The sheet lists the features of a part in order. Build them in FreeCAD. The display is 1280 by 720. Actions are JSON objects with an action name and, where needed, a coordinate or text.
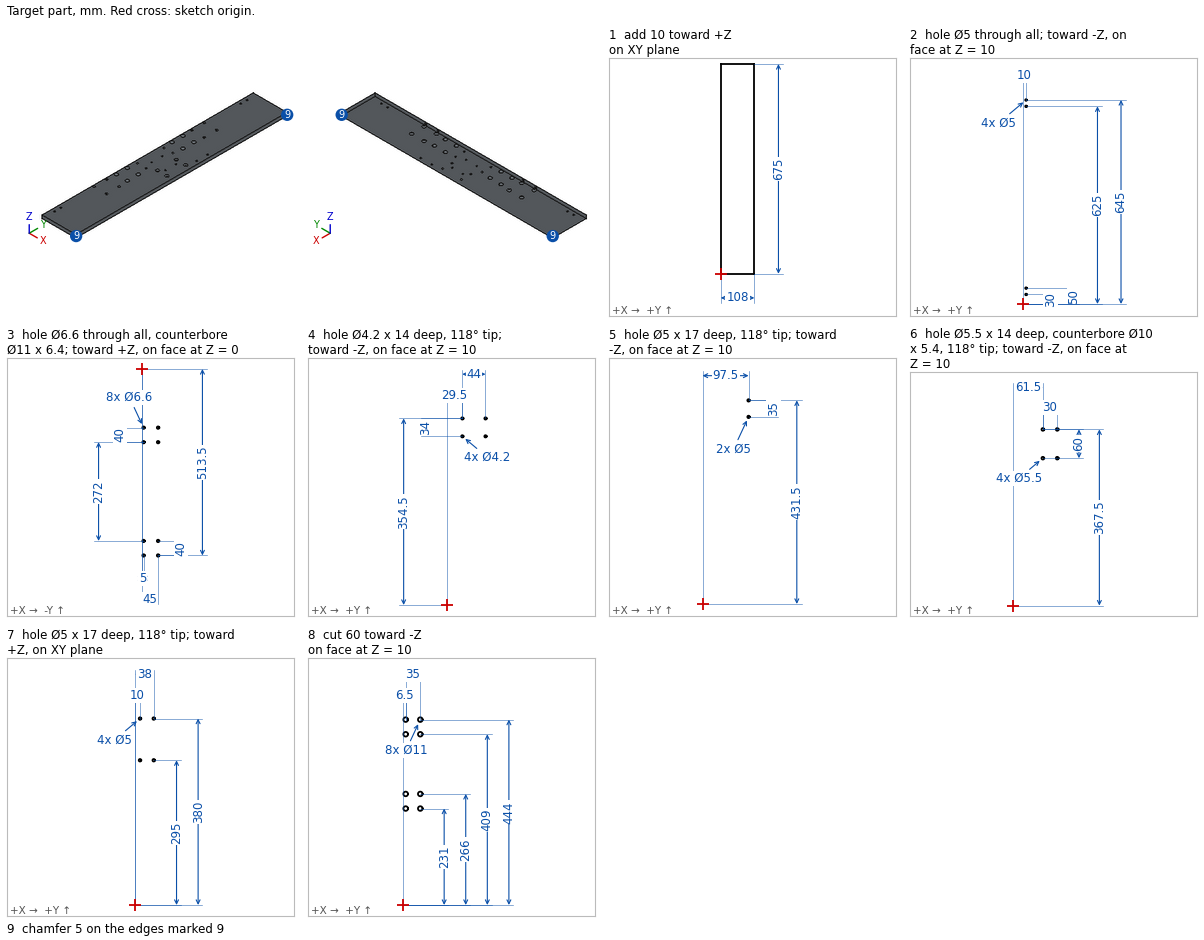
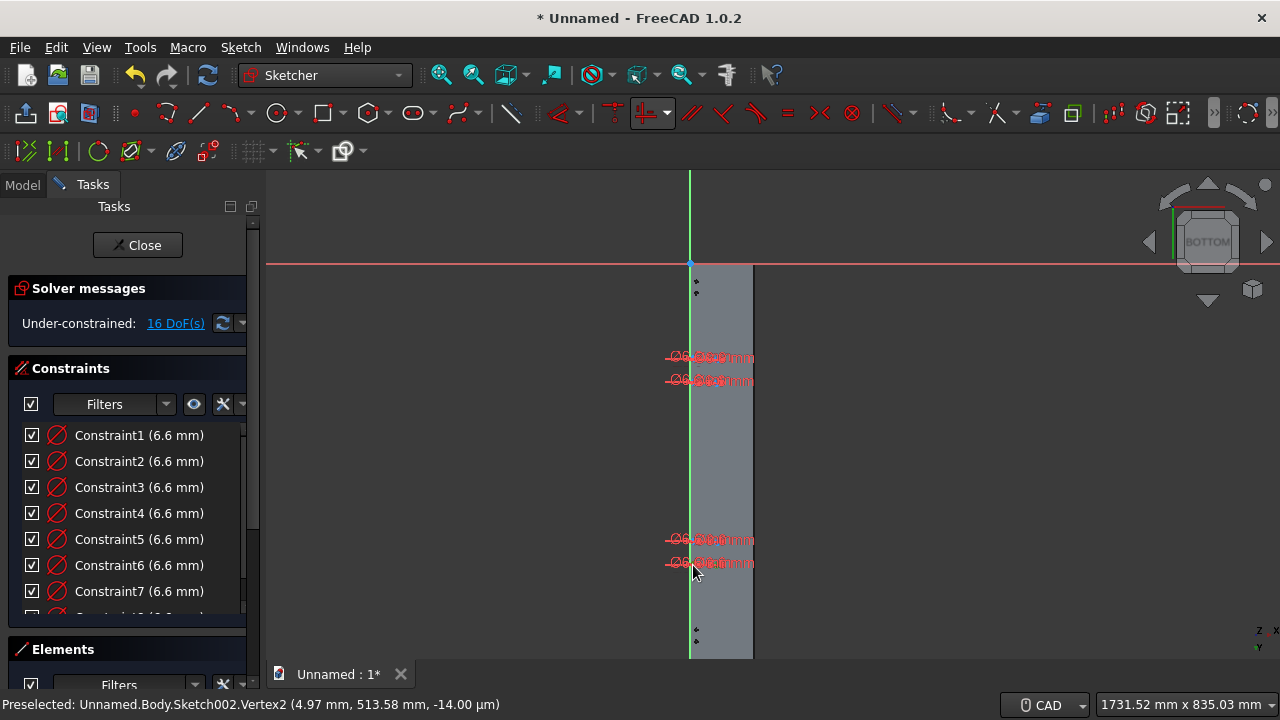
{"action": "key", "text": "h"}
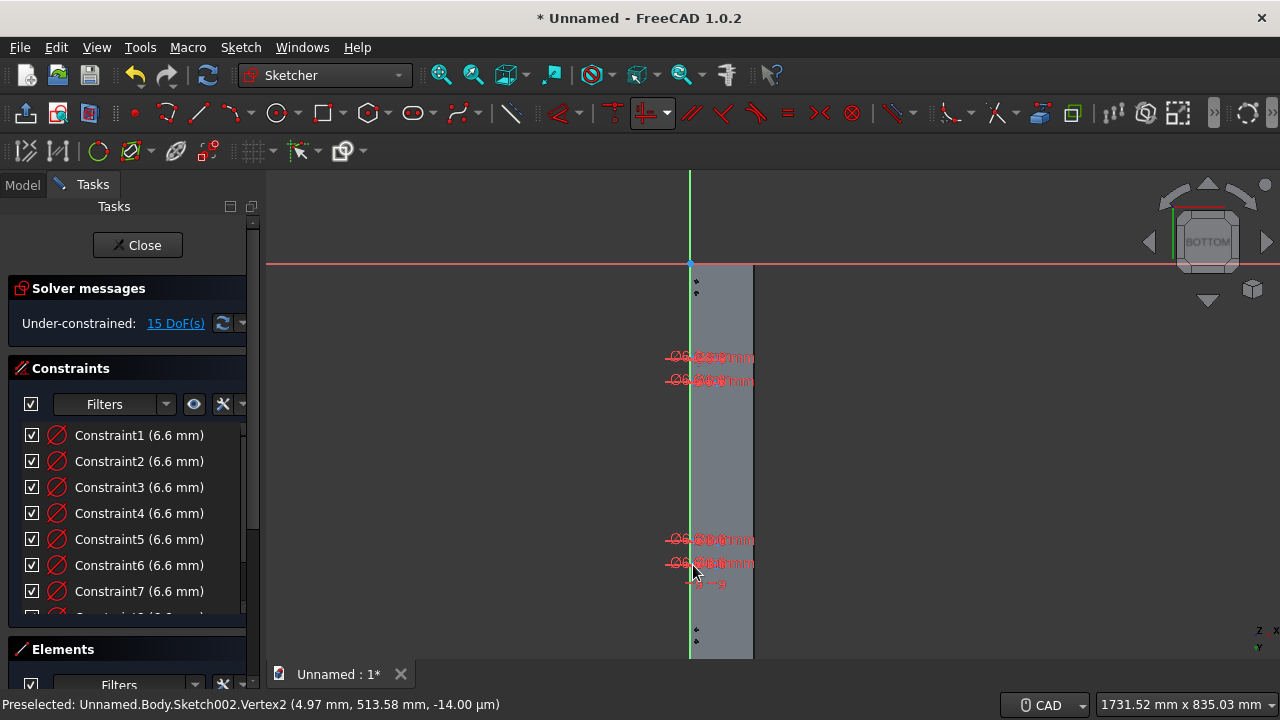
{"action": "left_click", "coordinate": [717, 565]}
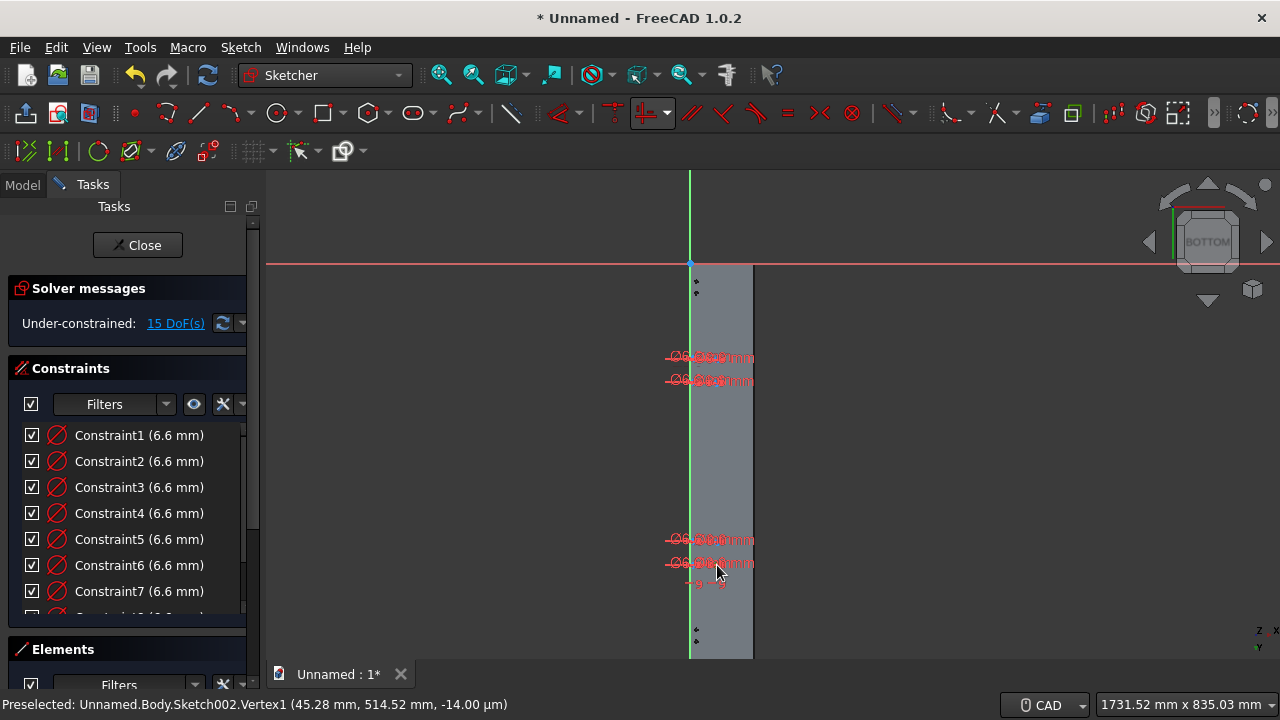
{"action": "left_click", "coordinate": [717, 542]}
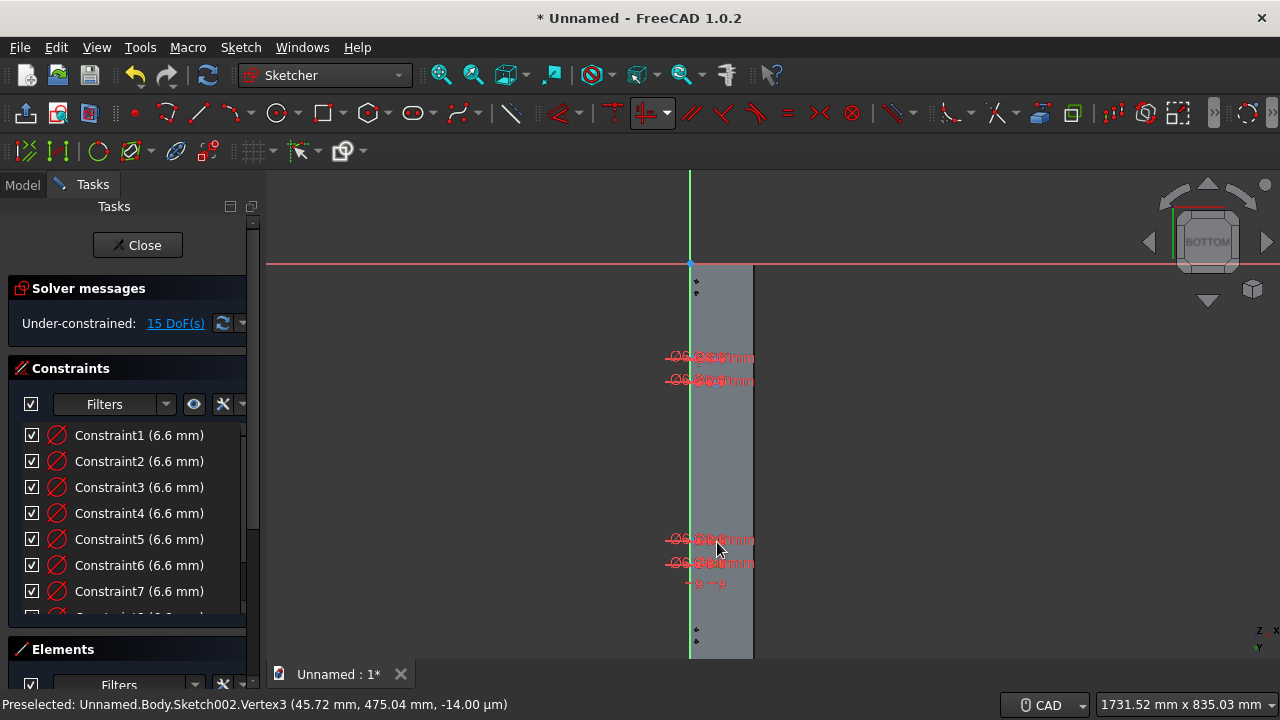
{"action": "key", "text": "v"}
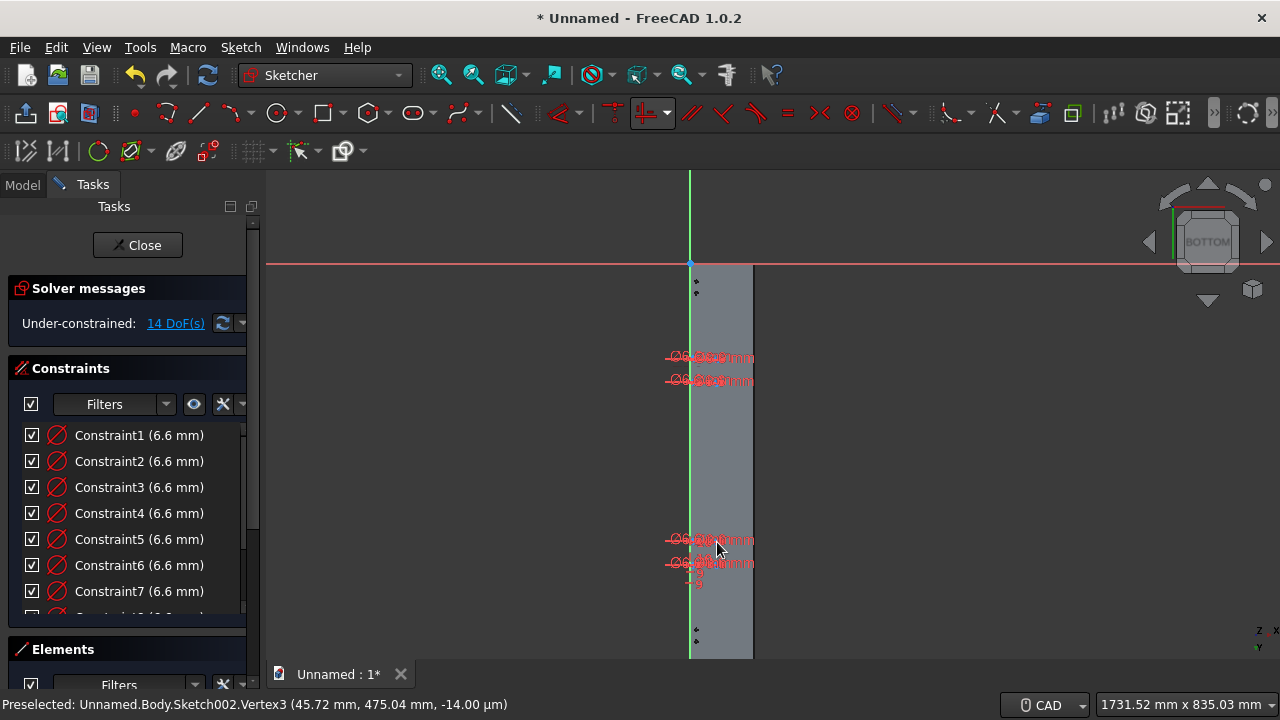
{"action": "left_click", "coordinate": [693, 565]}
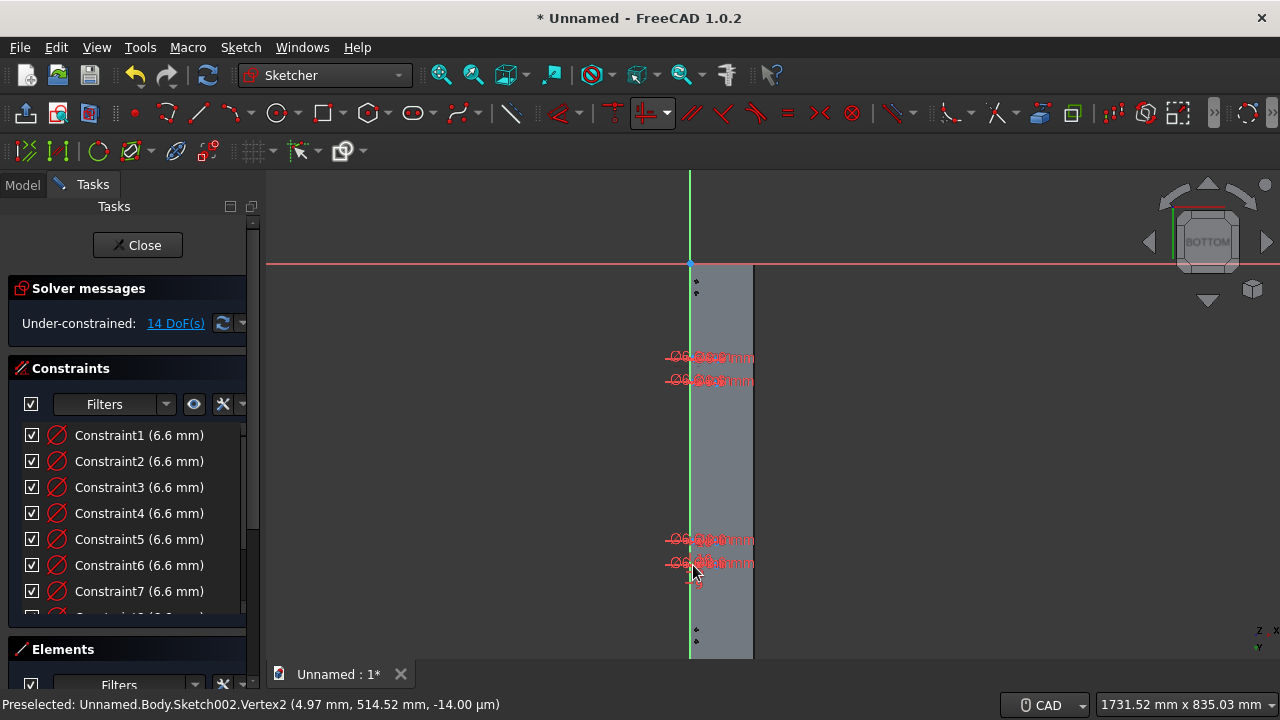
{"action": "scroll", "coordinate": [693, 541], "scroll_direction": "up", "scroll_amount": 4}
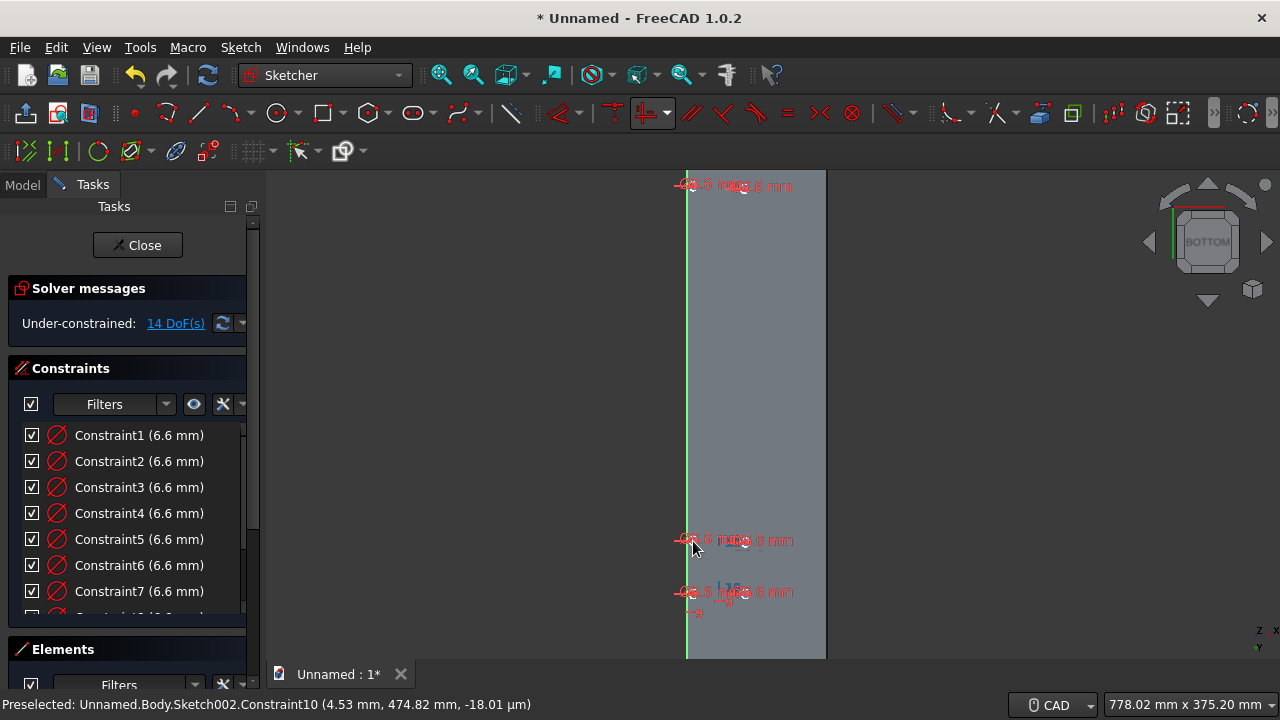
{"action": "left_click", "coordinate": [693, 541]}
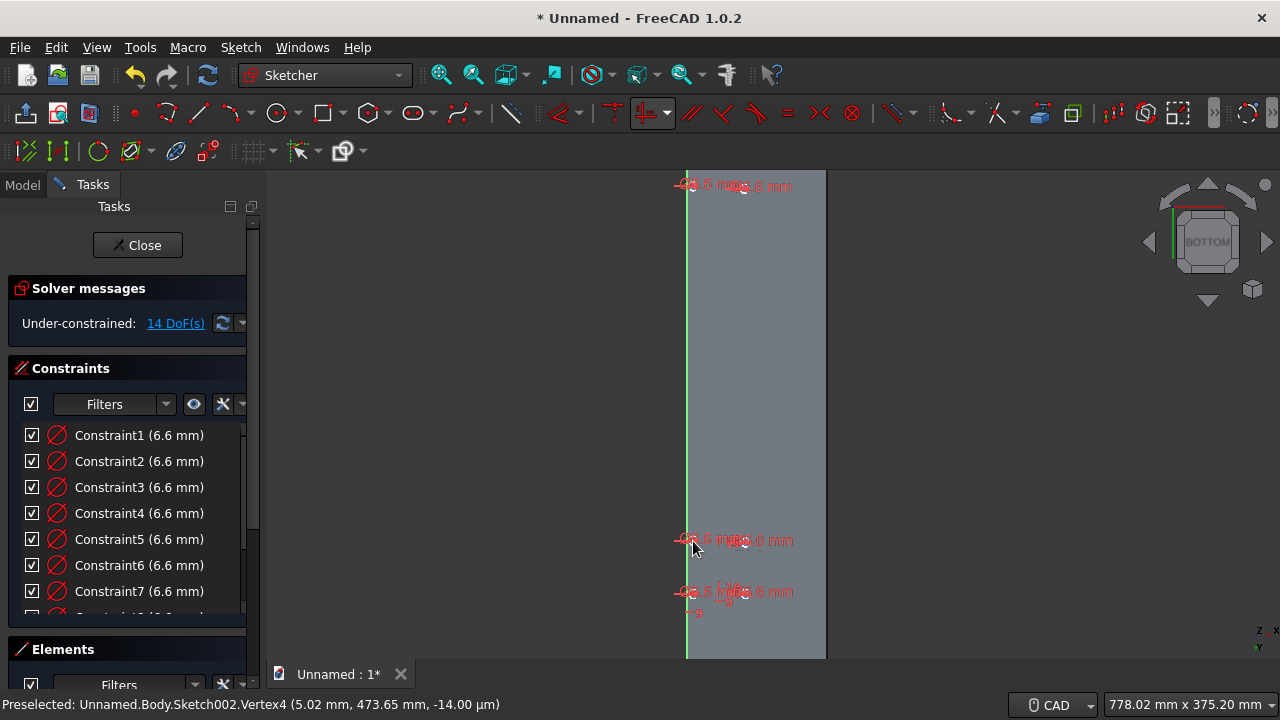
{"action": "key", "text": "v"}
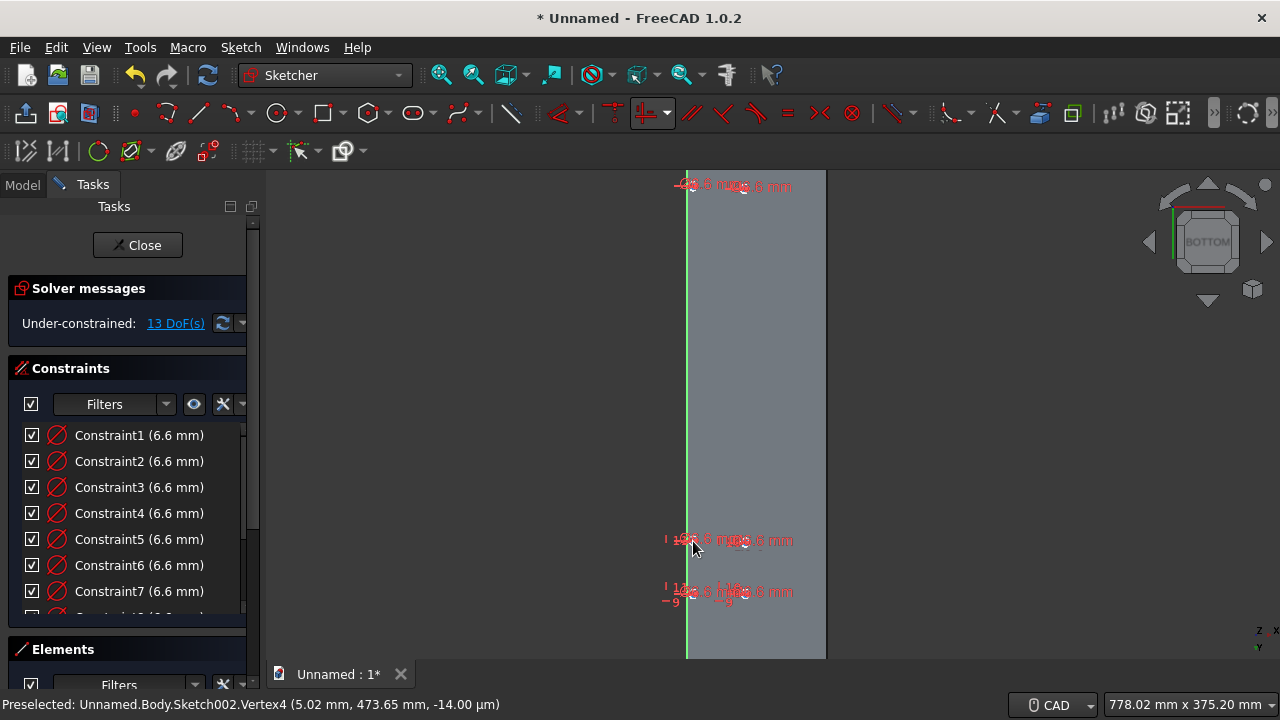
{"action": "left_click", "coordinate": [746, 543]}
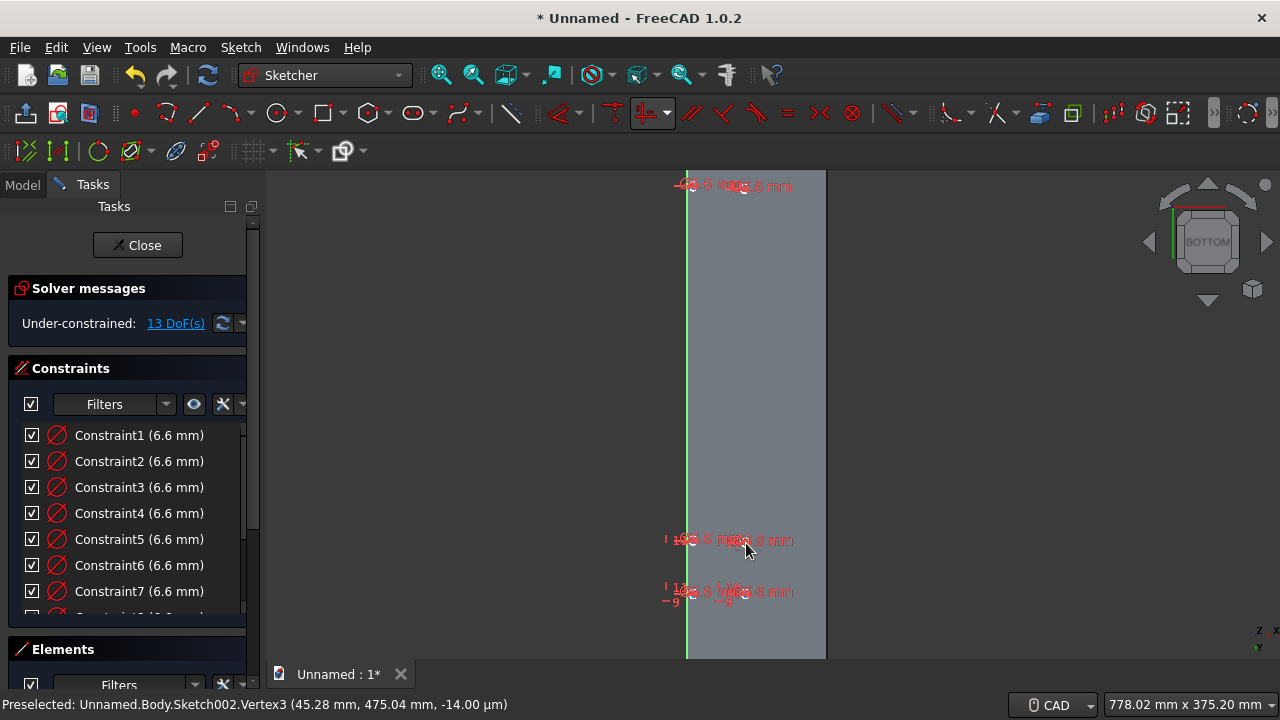
{"action": "left_click", "coordinate": [693, 541]}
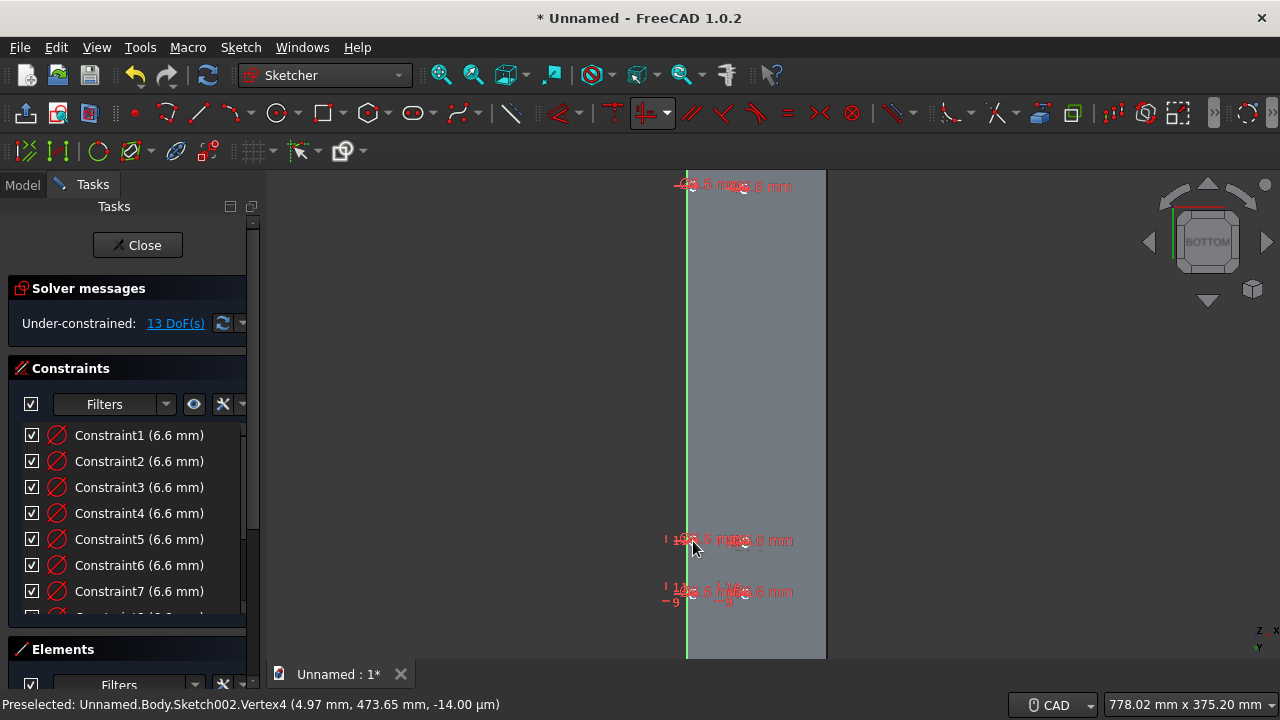
{"action": "left_click", "coordinate": [670, 114]}